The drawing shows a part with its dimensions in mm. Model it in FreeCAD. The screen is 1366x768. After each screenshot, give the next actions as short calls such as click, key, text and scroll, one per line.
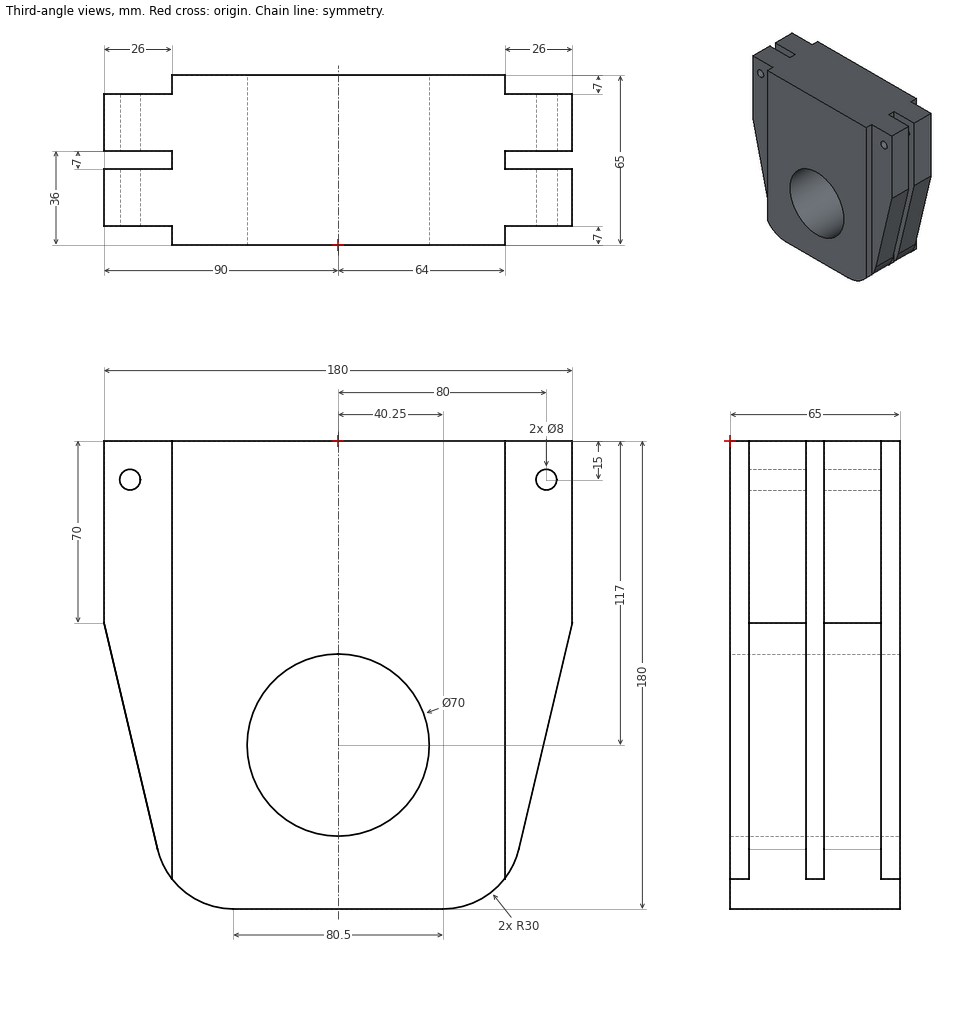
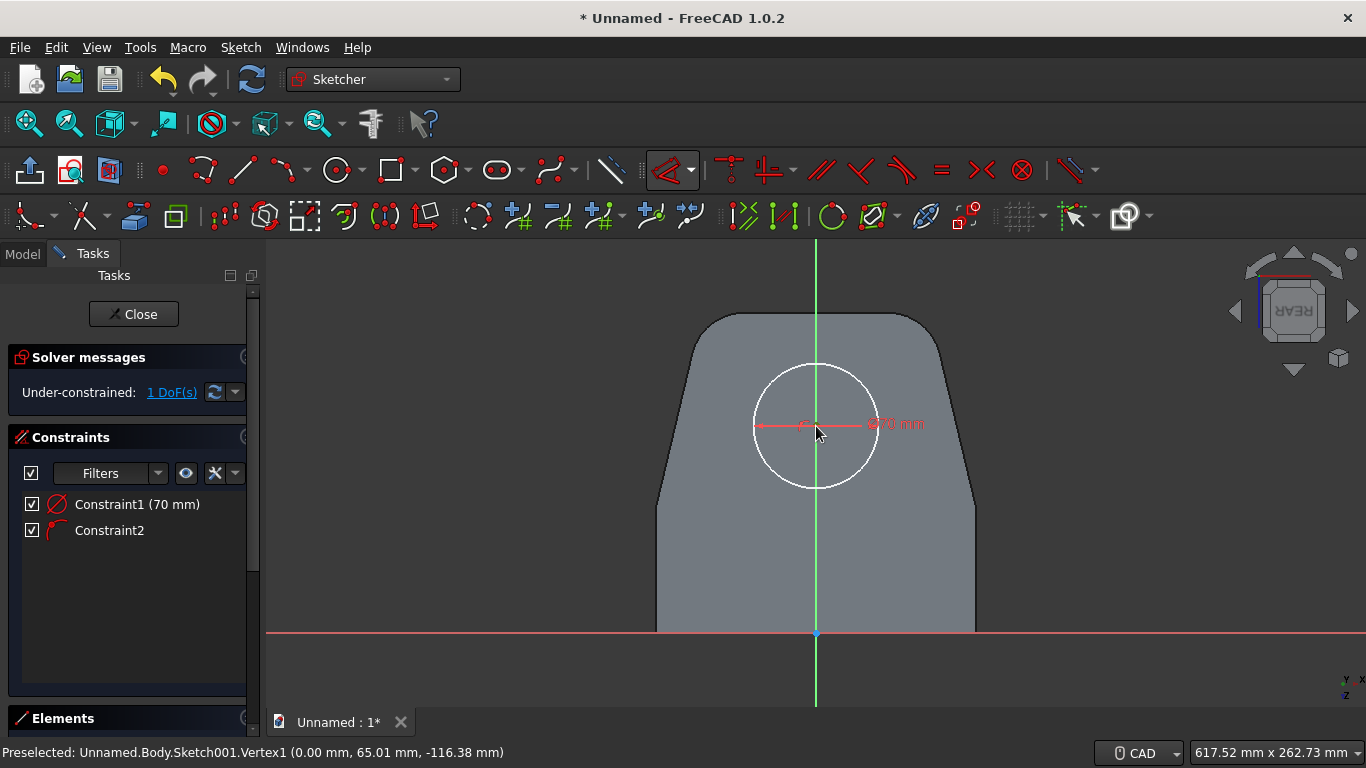
key(i)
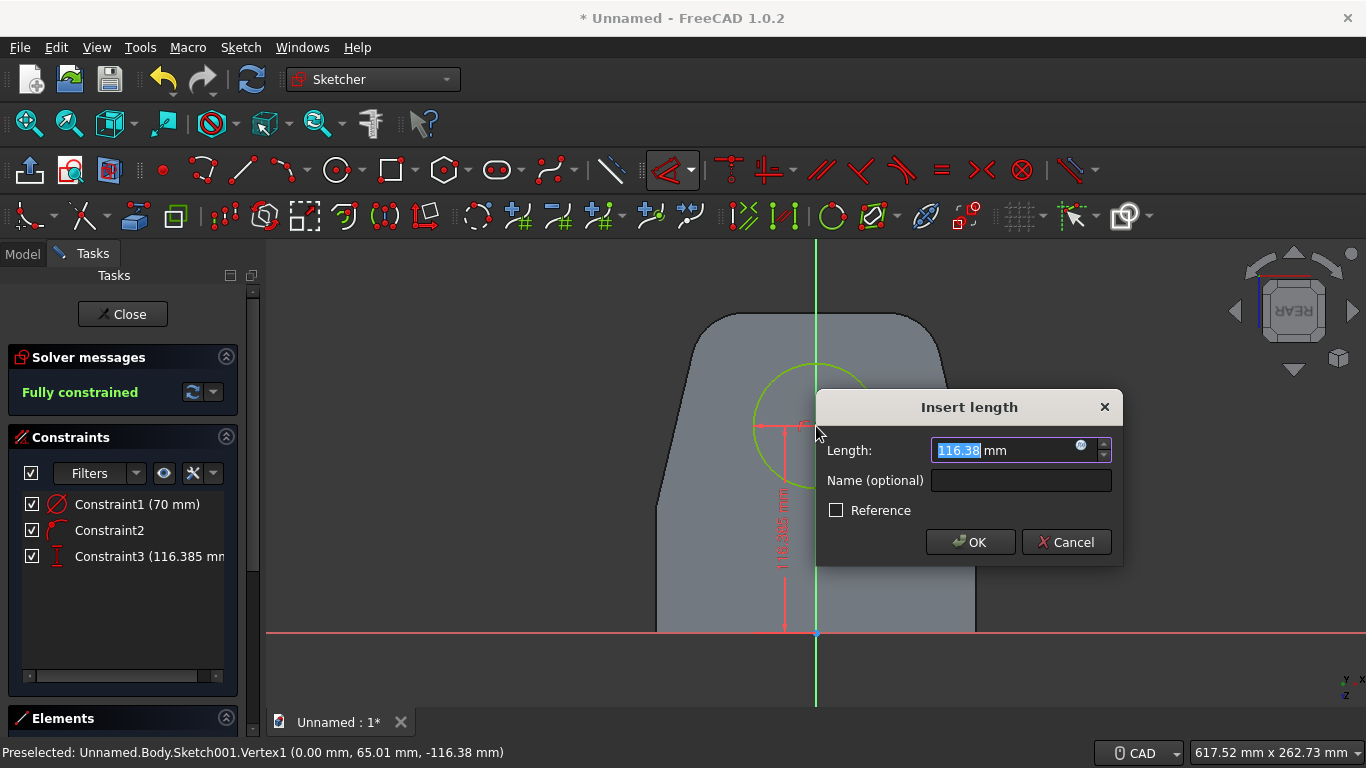
text(117)
key(Return)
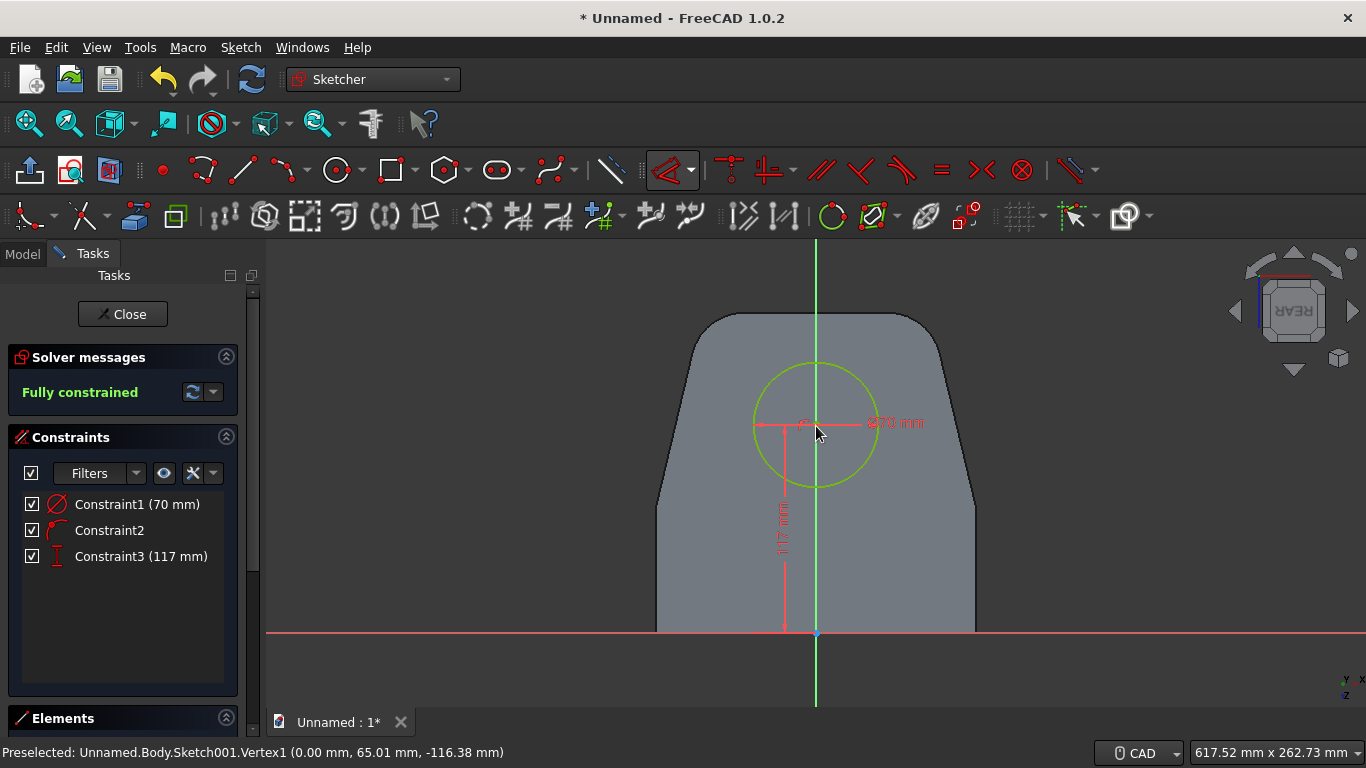
click(123, 314)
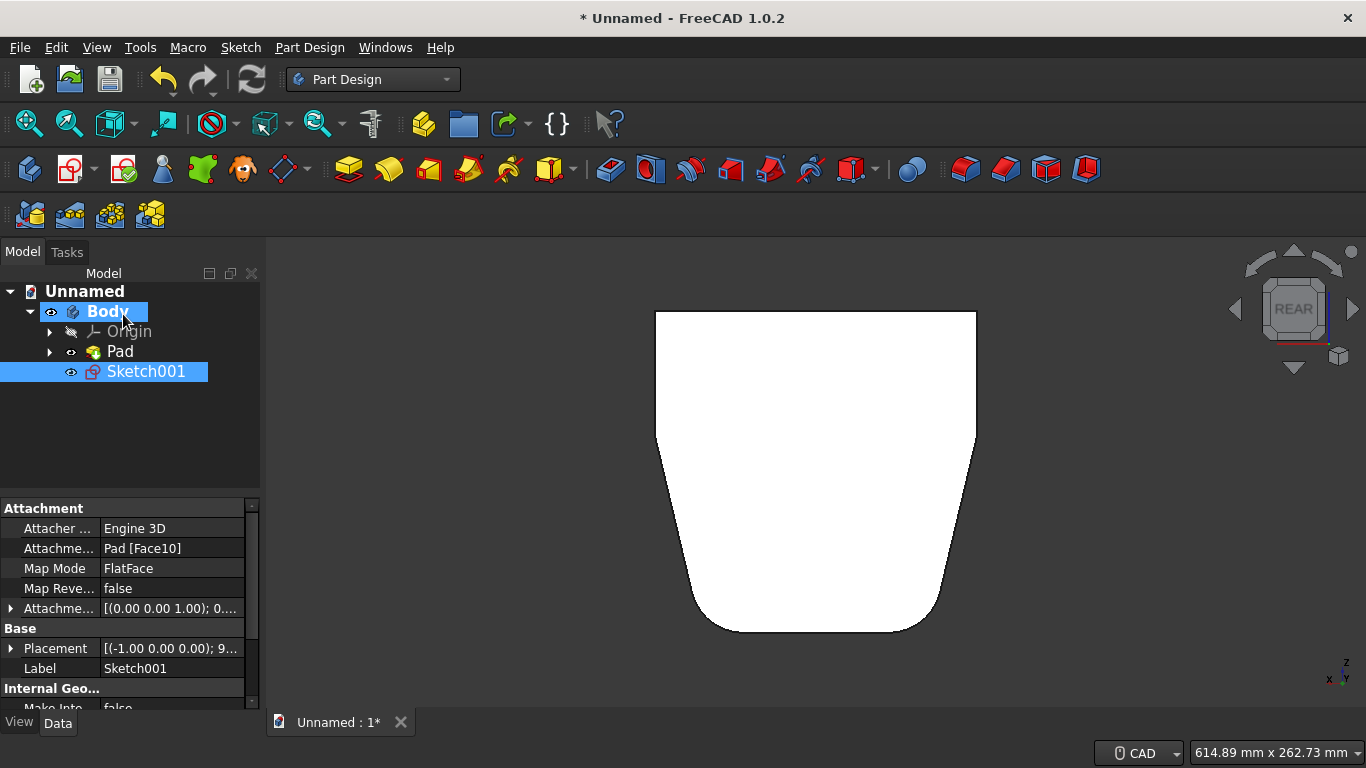
click(612, 170)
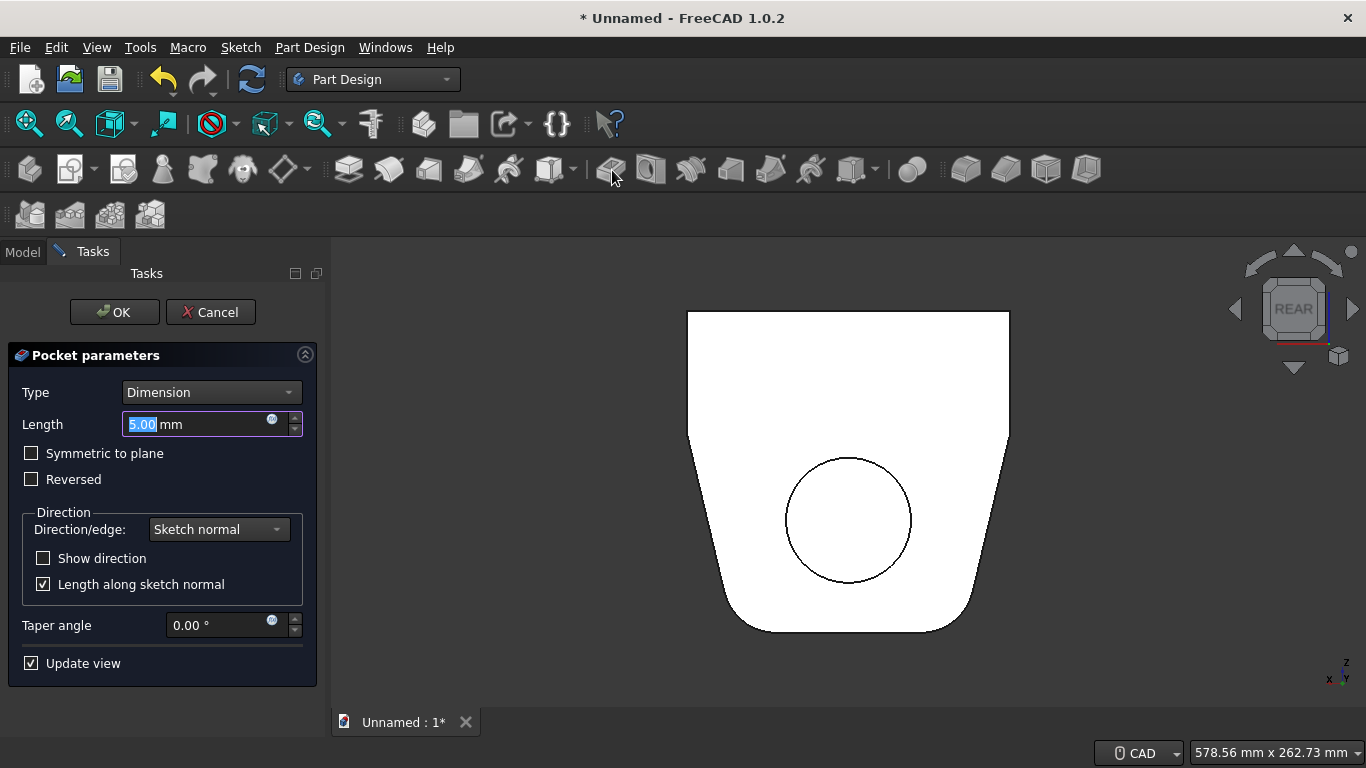
text(65)
key(Tab)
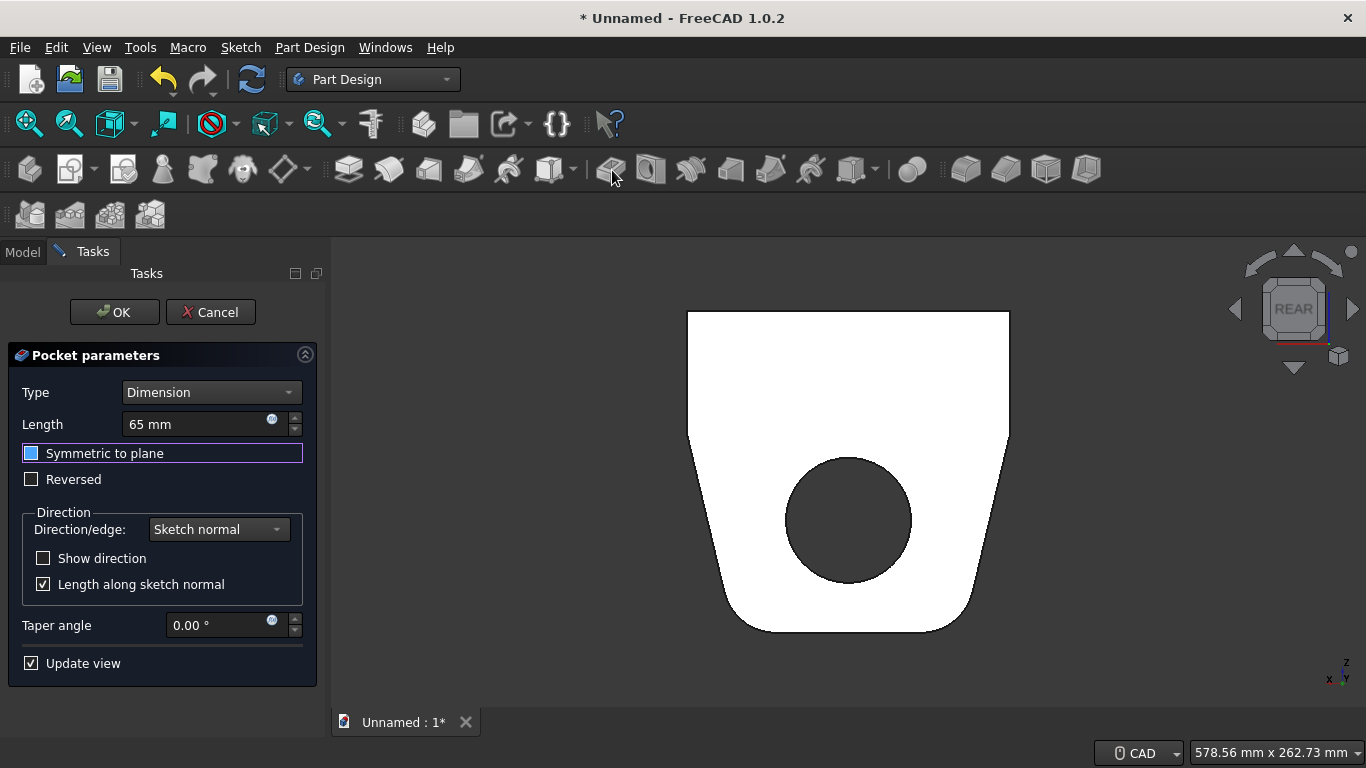
click(115, 312)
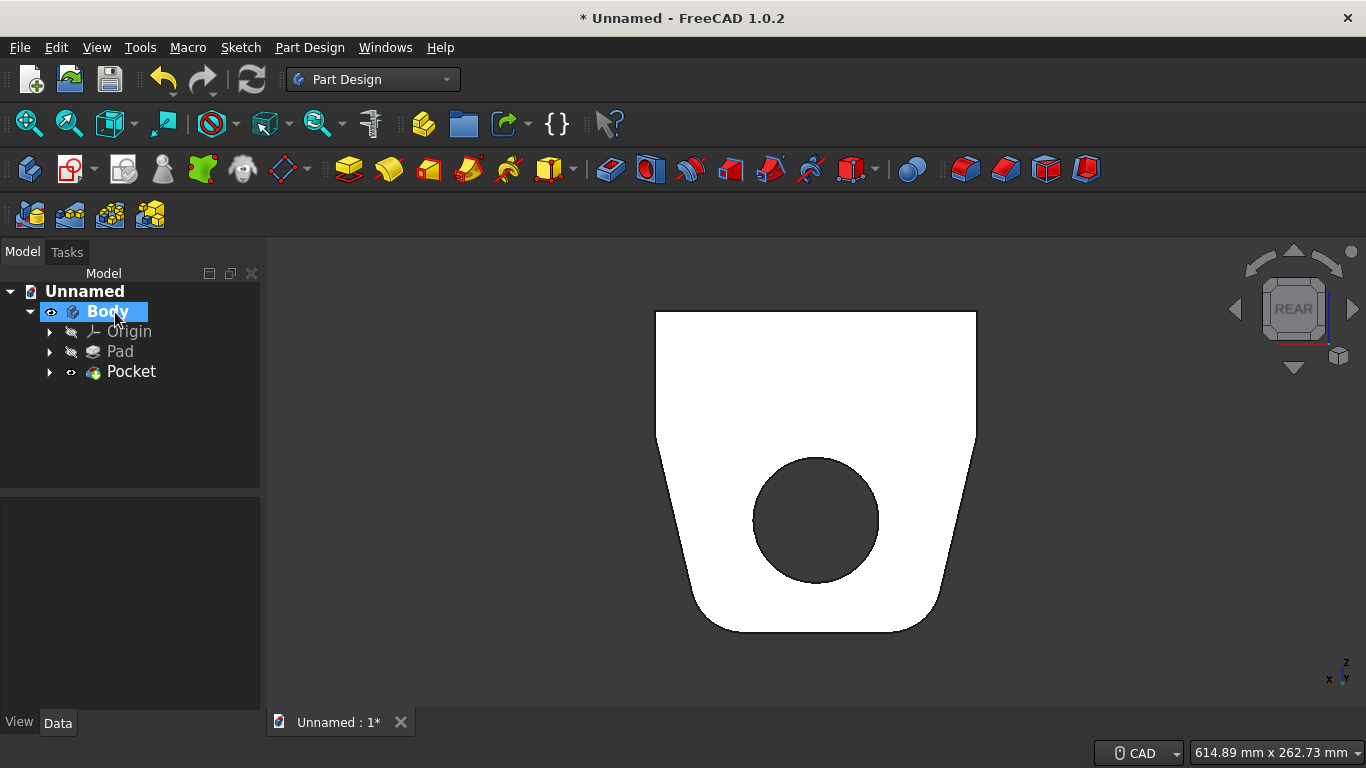
click(70, 170)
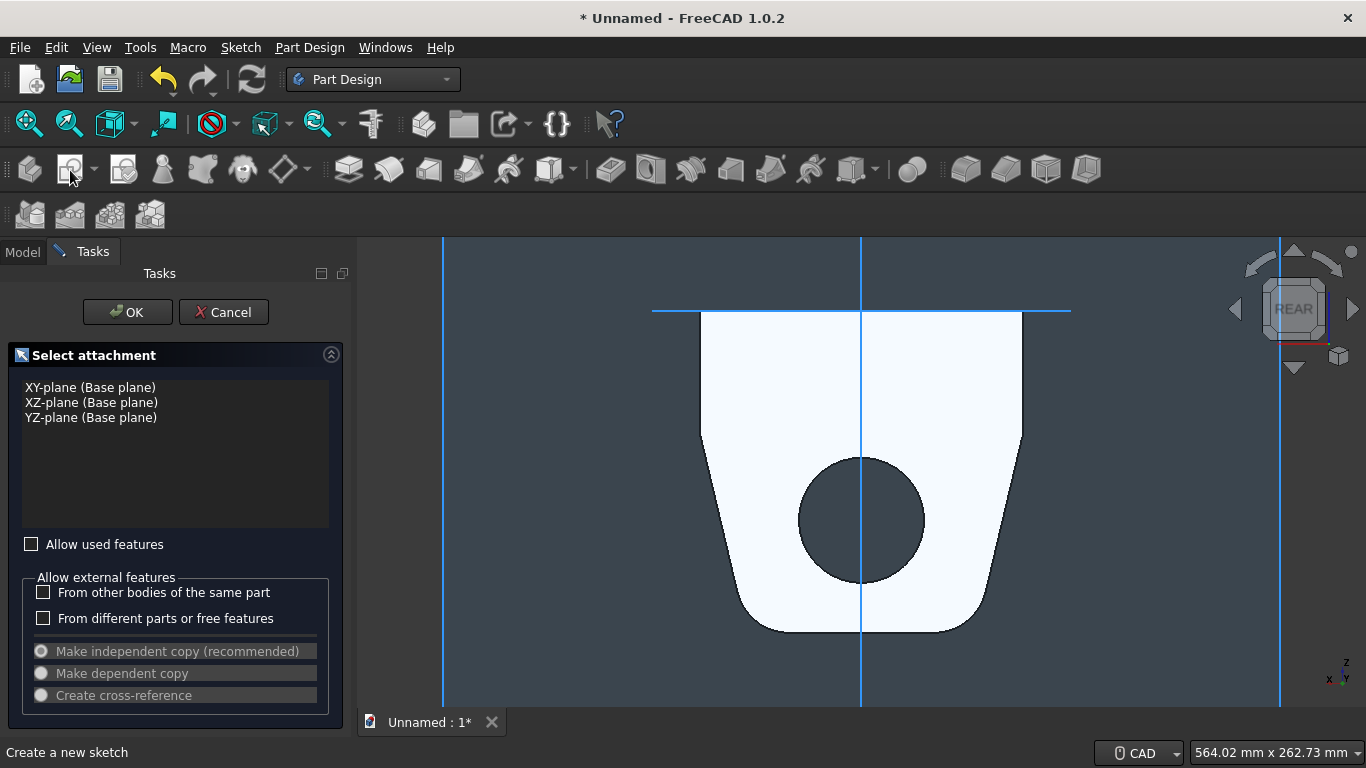
click(82, 388)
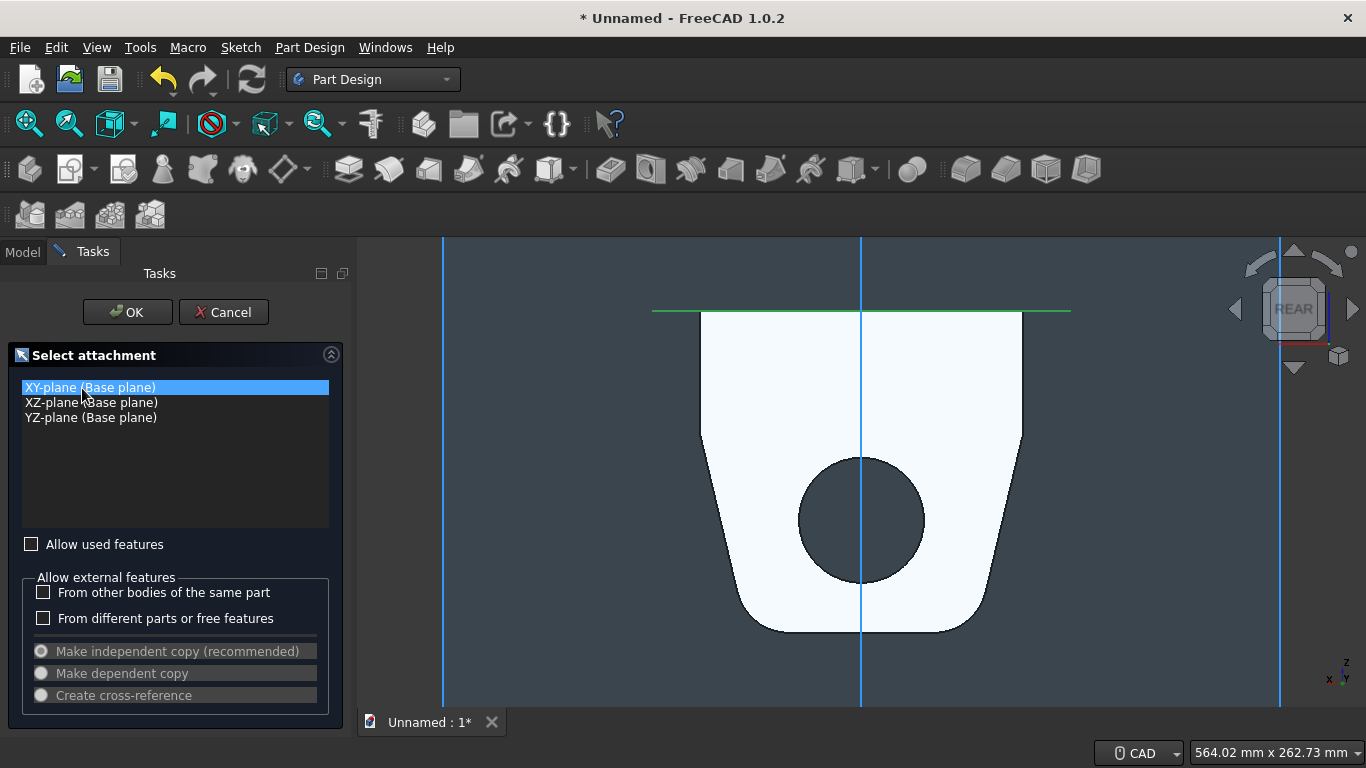
click(128, 312)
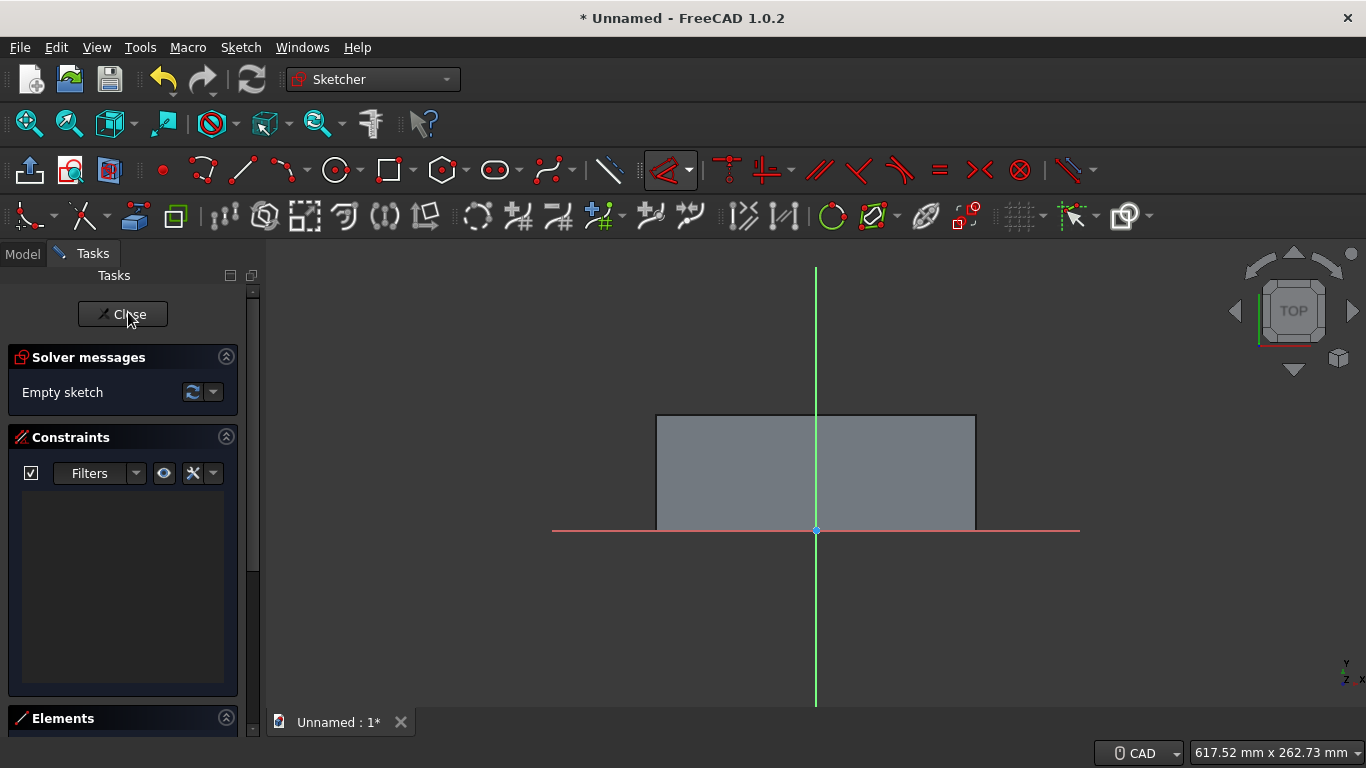
scroll(899, 473, up, 3)